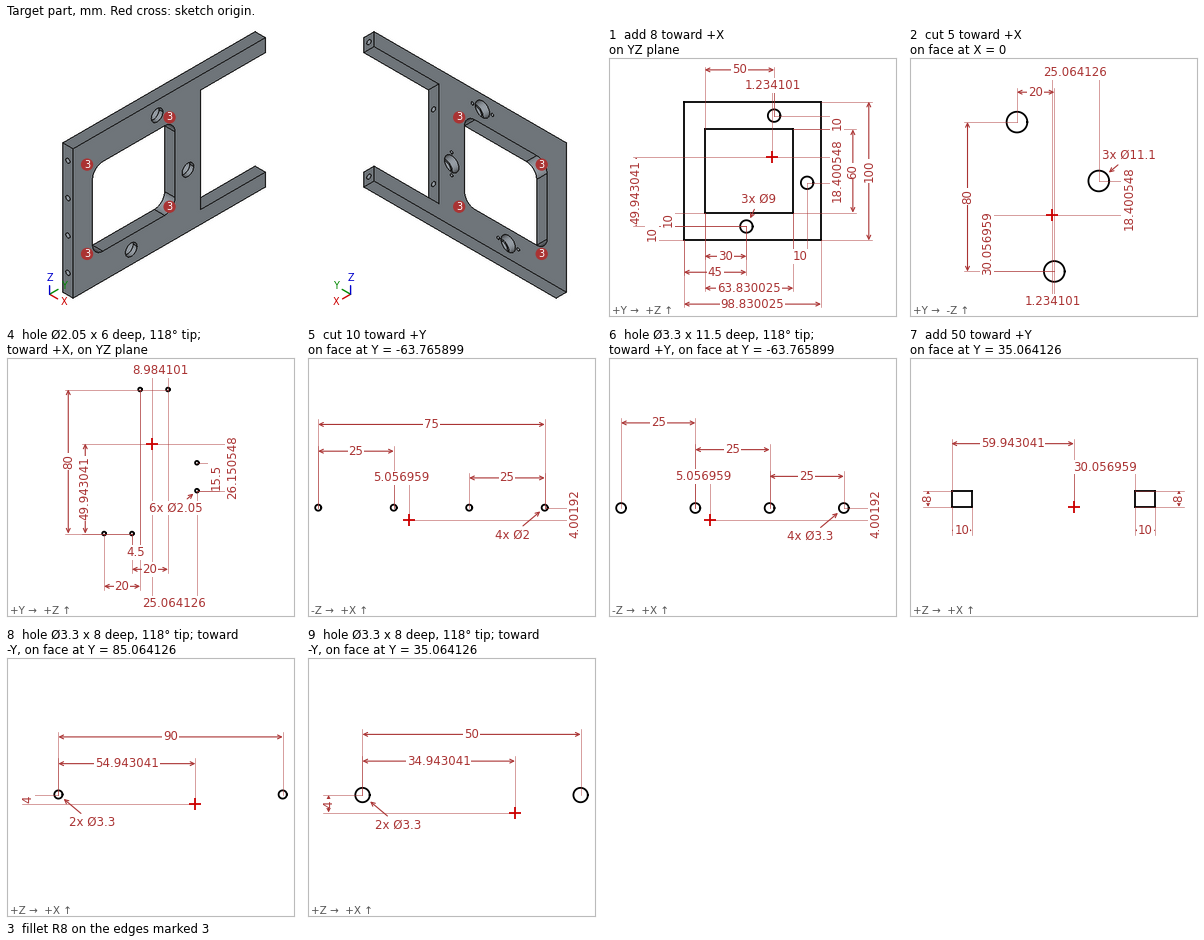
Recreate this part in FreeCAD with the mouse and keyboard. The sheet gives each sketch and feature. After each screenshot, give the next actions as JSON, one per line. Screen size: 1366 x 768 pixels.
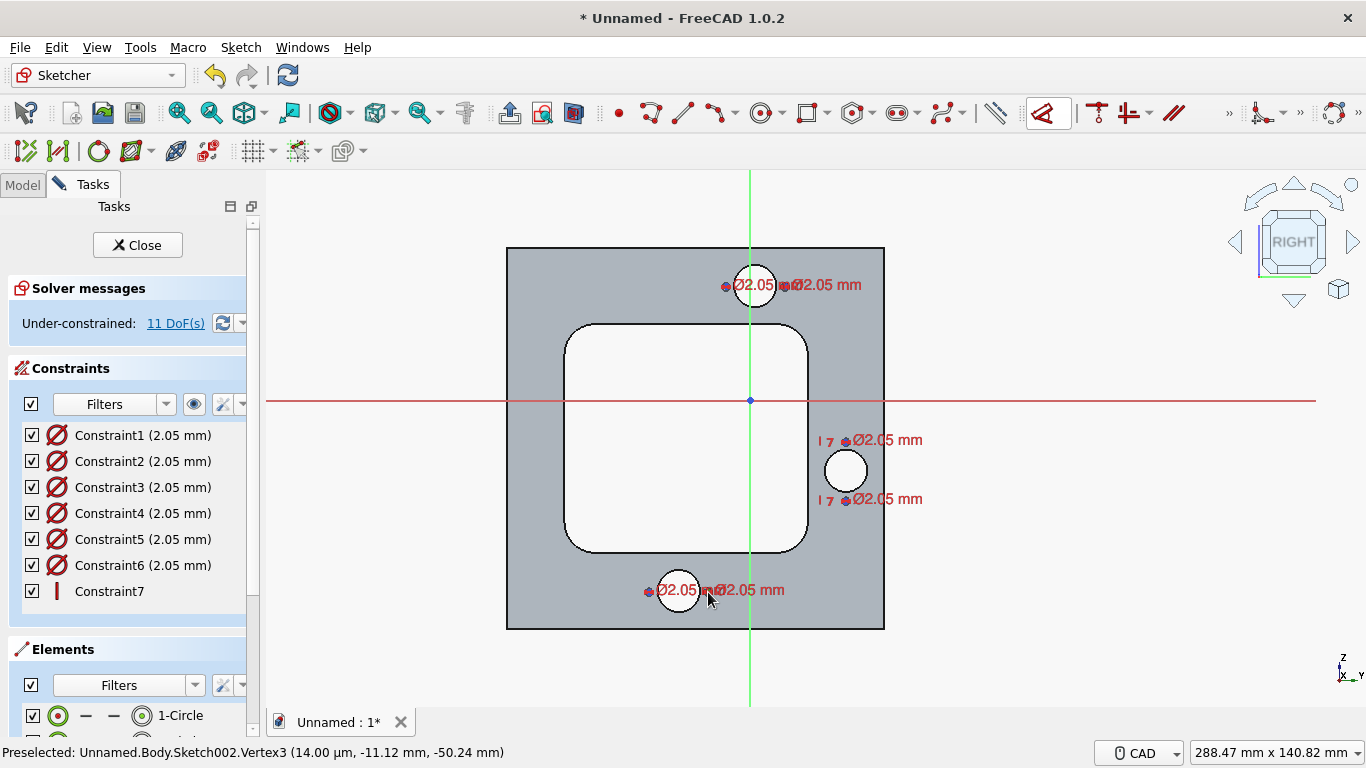
{"action": "left_click", "coordinate": [649, 592]}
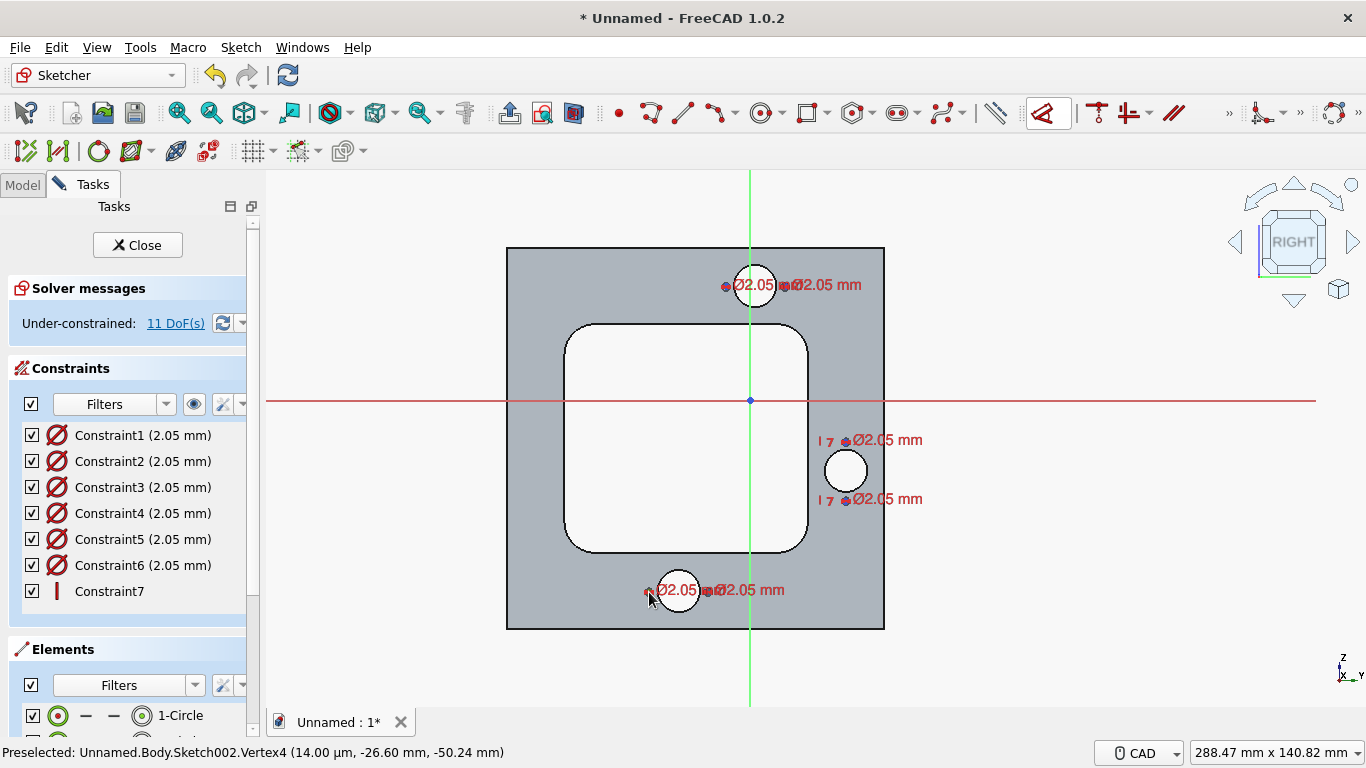
{"action": "key", "text": "h"}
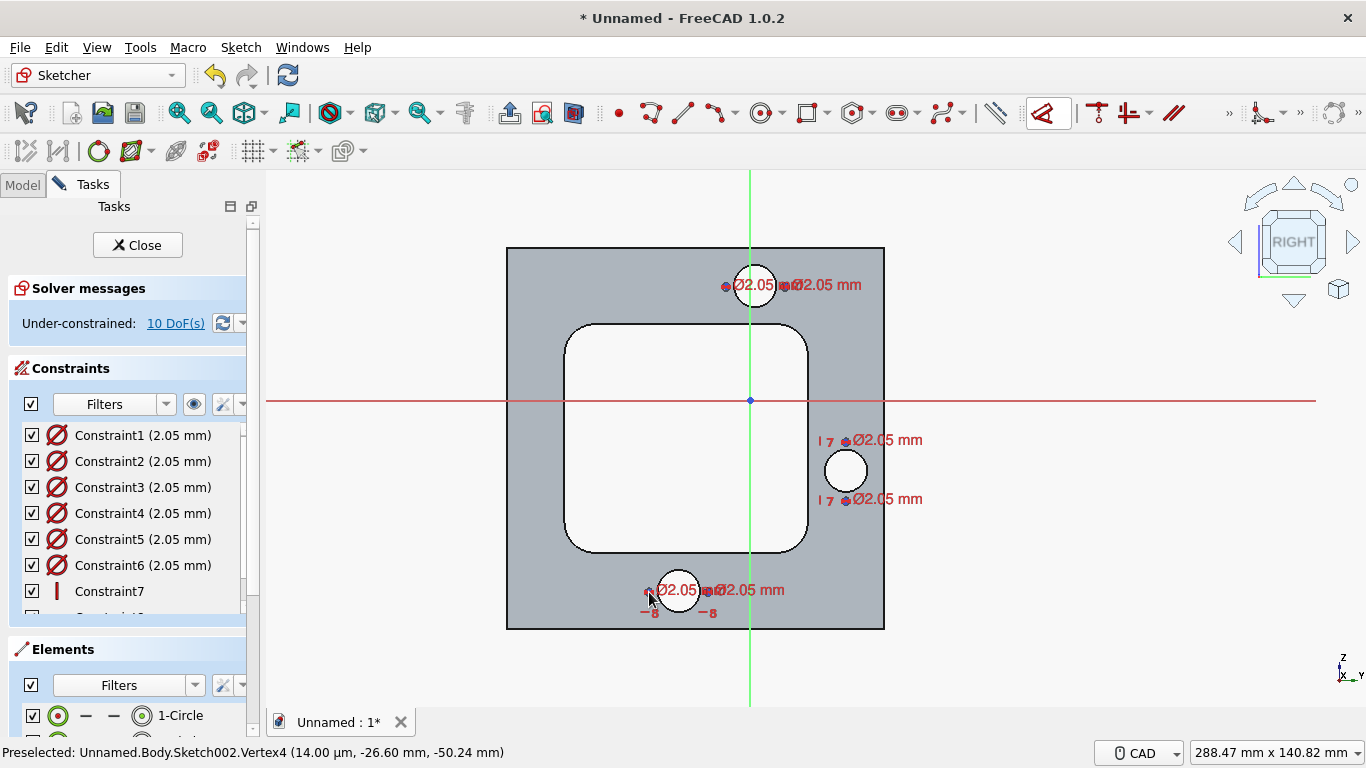
{"action": "left_click", "coordinate": [785, 287]}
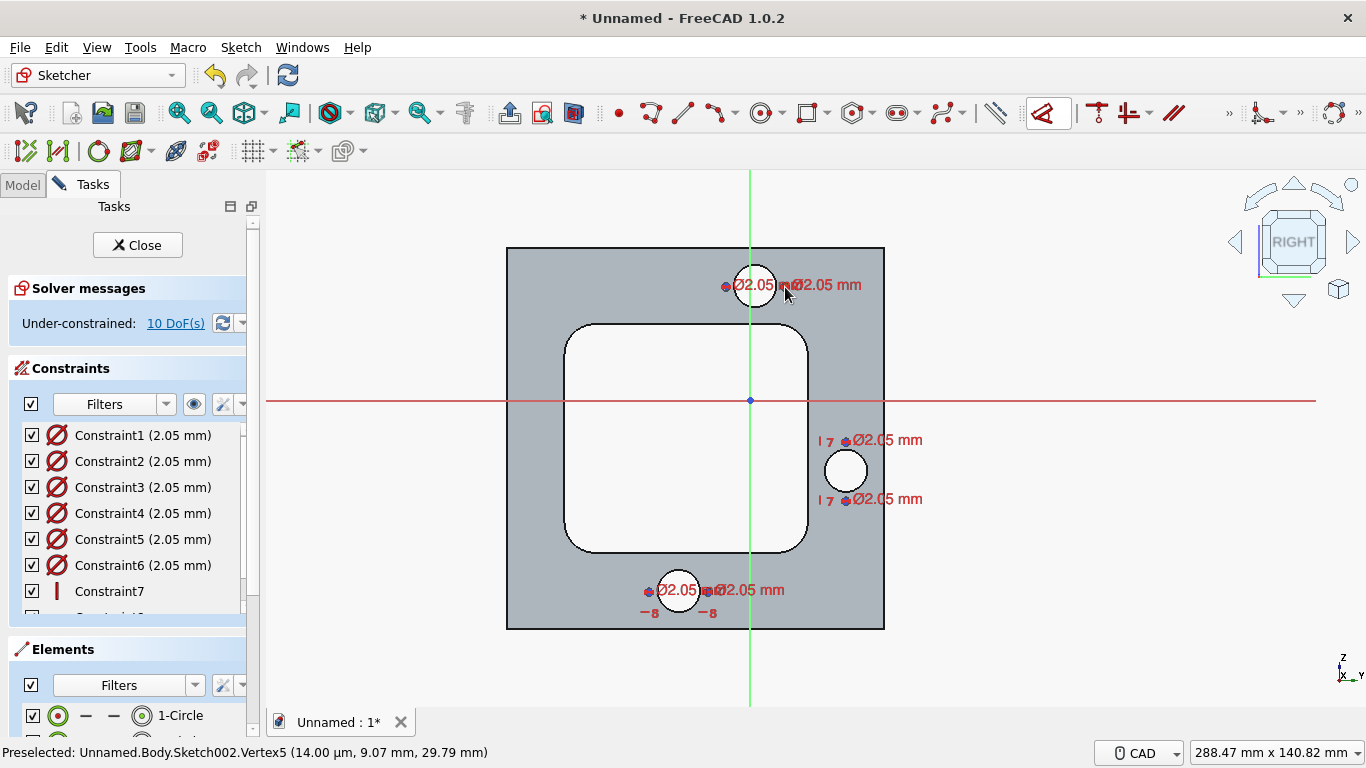
{"action": "left_click", "coordinate": [726, 287]}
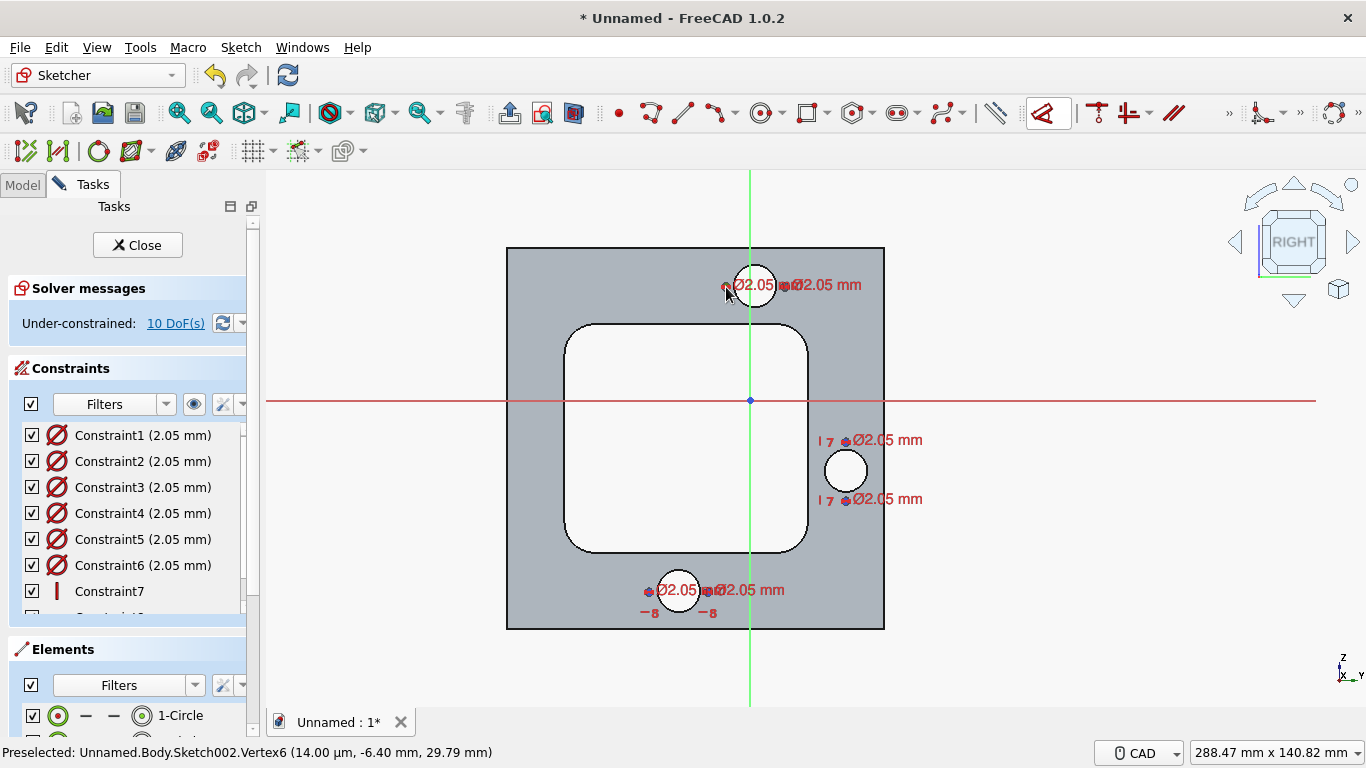
{"action": "key", "text": "h"}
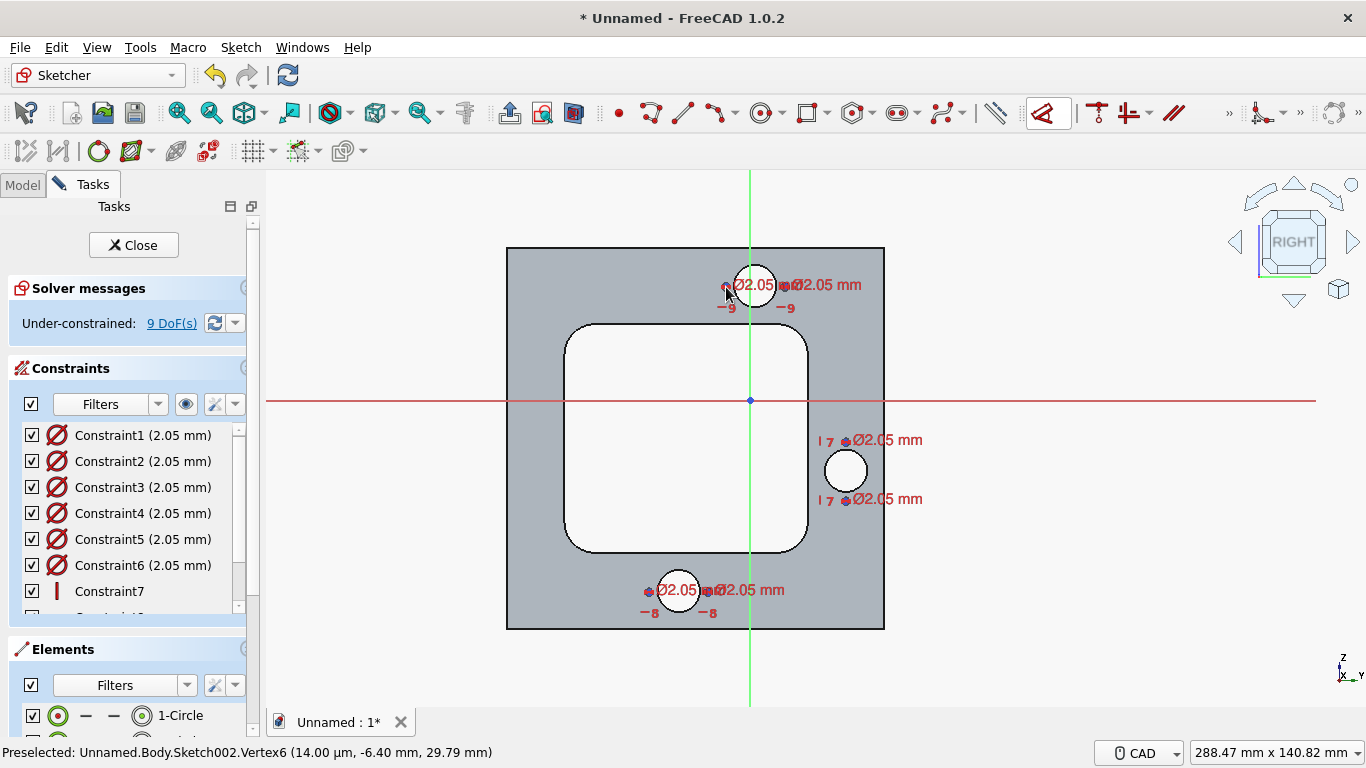
{"action": "left_click", "coordinate": [708, 592]}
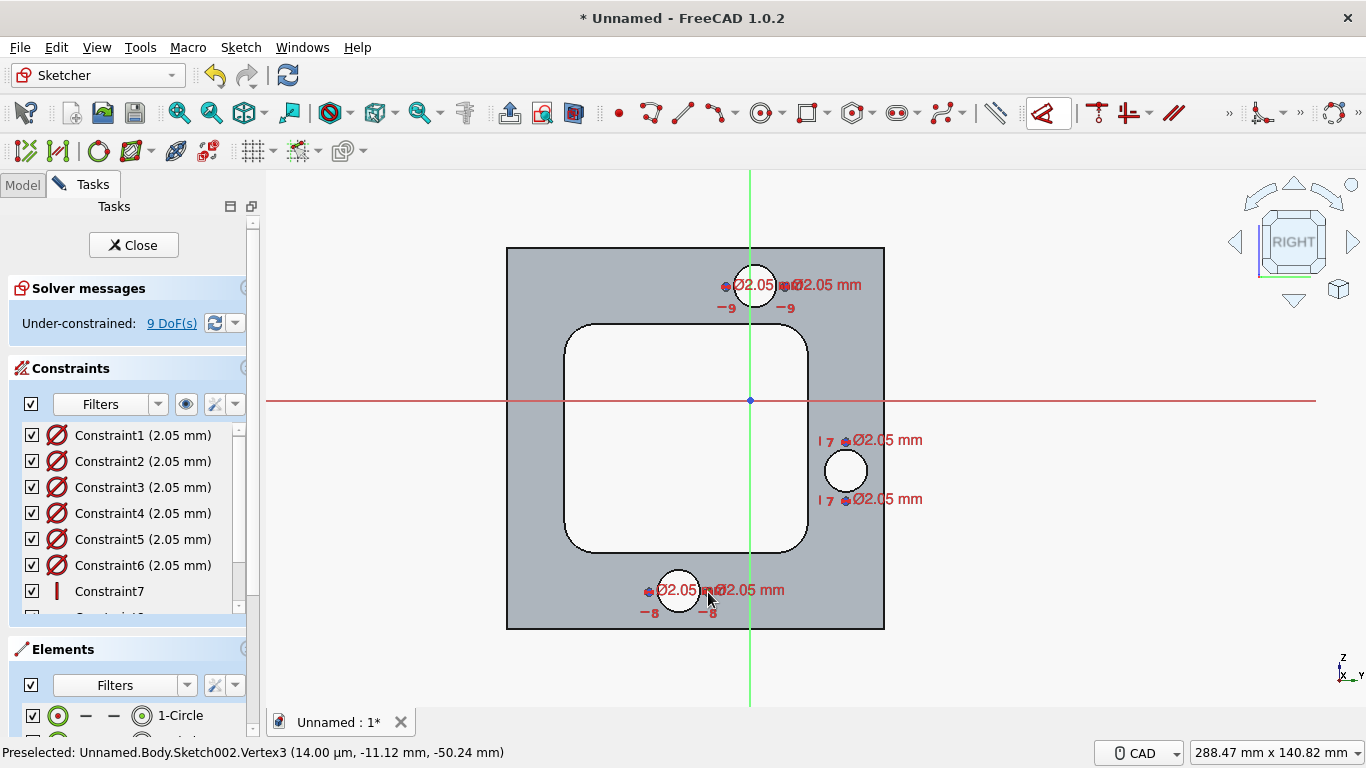
{"action": "left_click", "coordinate": [785, 287]}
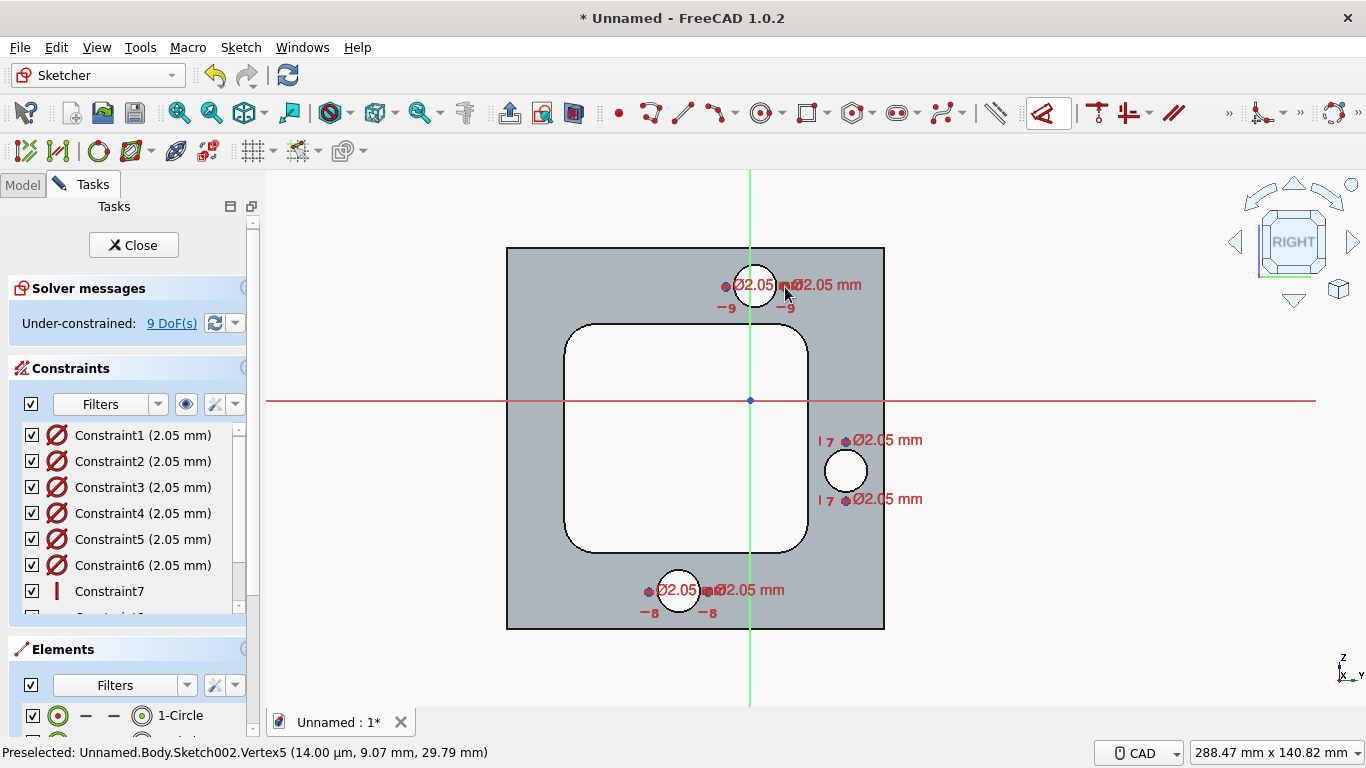
{"action": "key", "text": "l"}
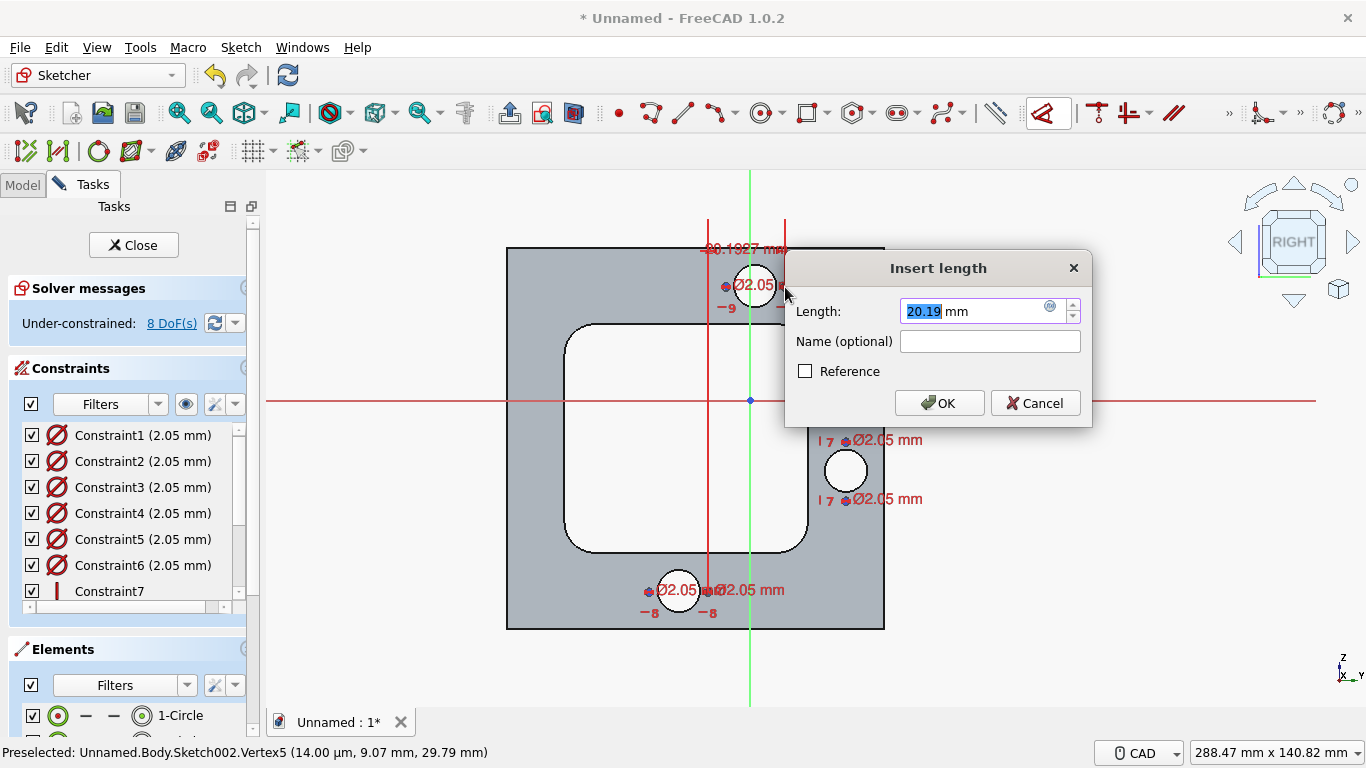
{"action": "type", "text": "20"}
{"action": "key", "text": "Return"}